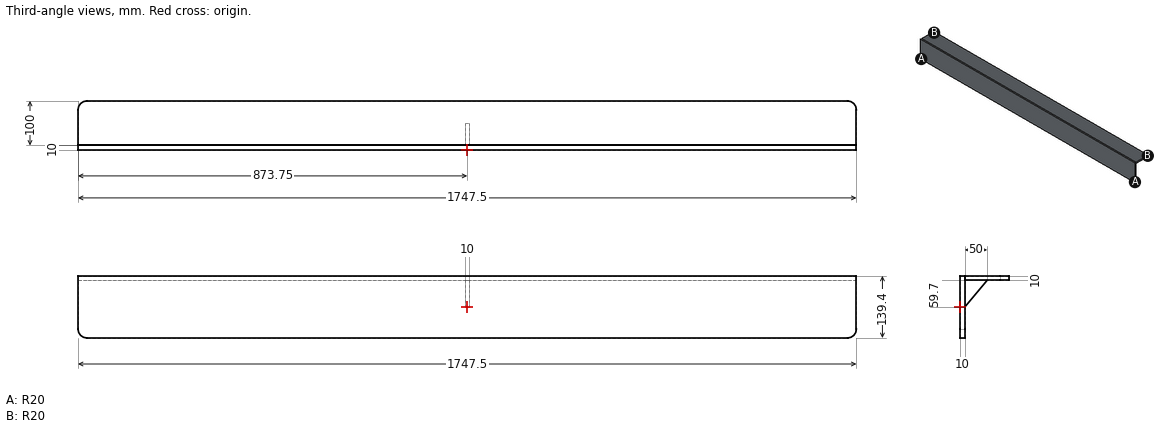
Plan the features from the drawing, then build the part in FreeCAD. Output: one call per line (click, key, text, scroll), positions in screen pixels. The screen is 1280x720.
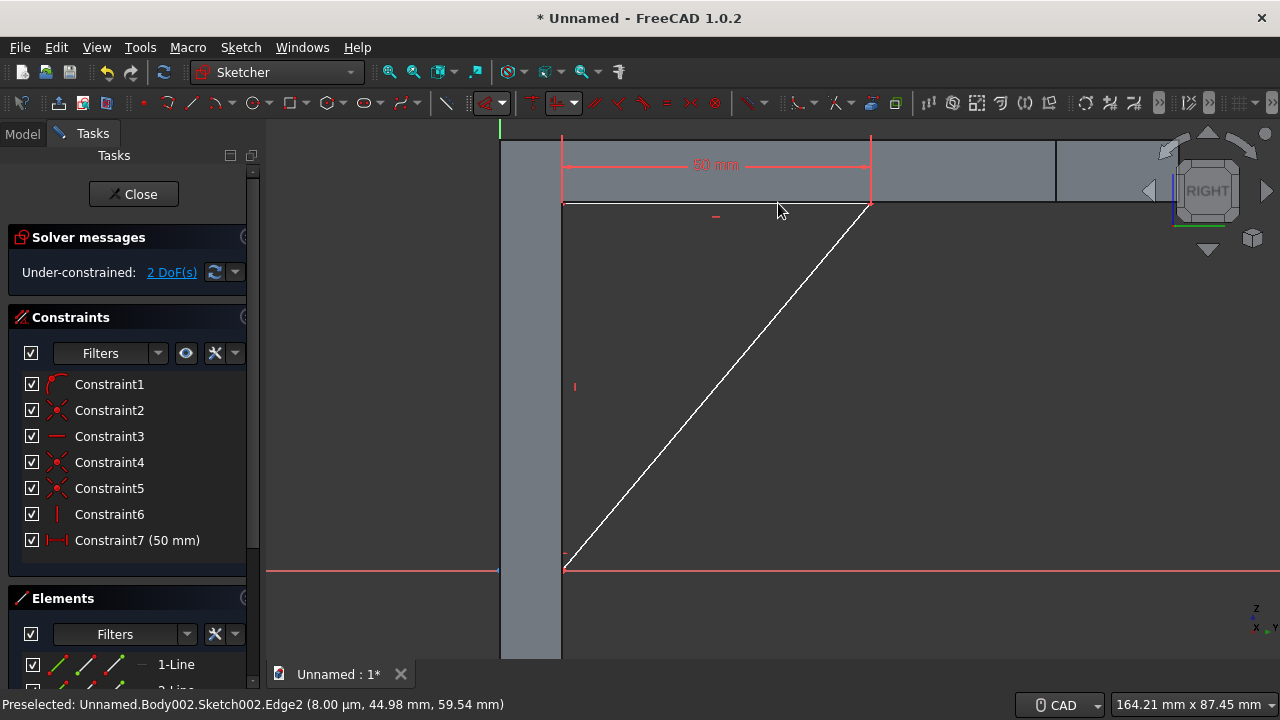
click(562, 571)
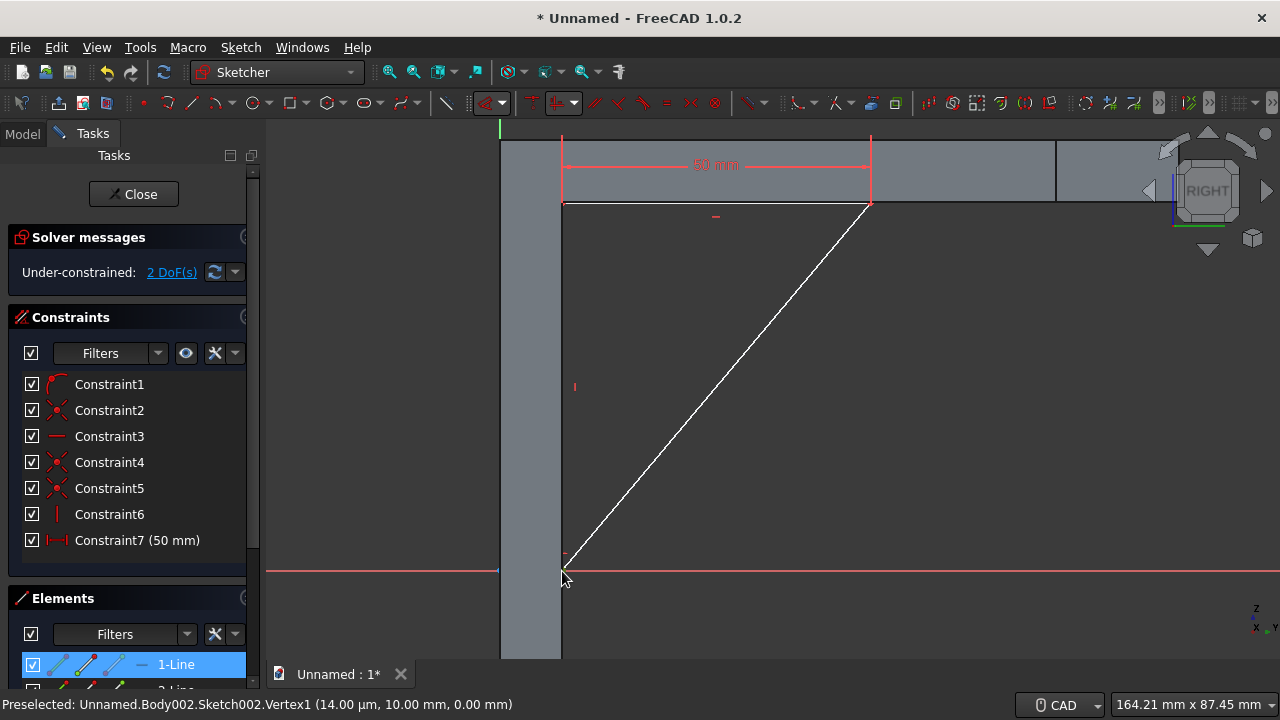
key(l)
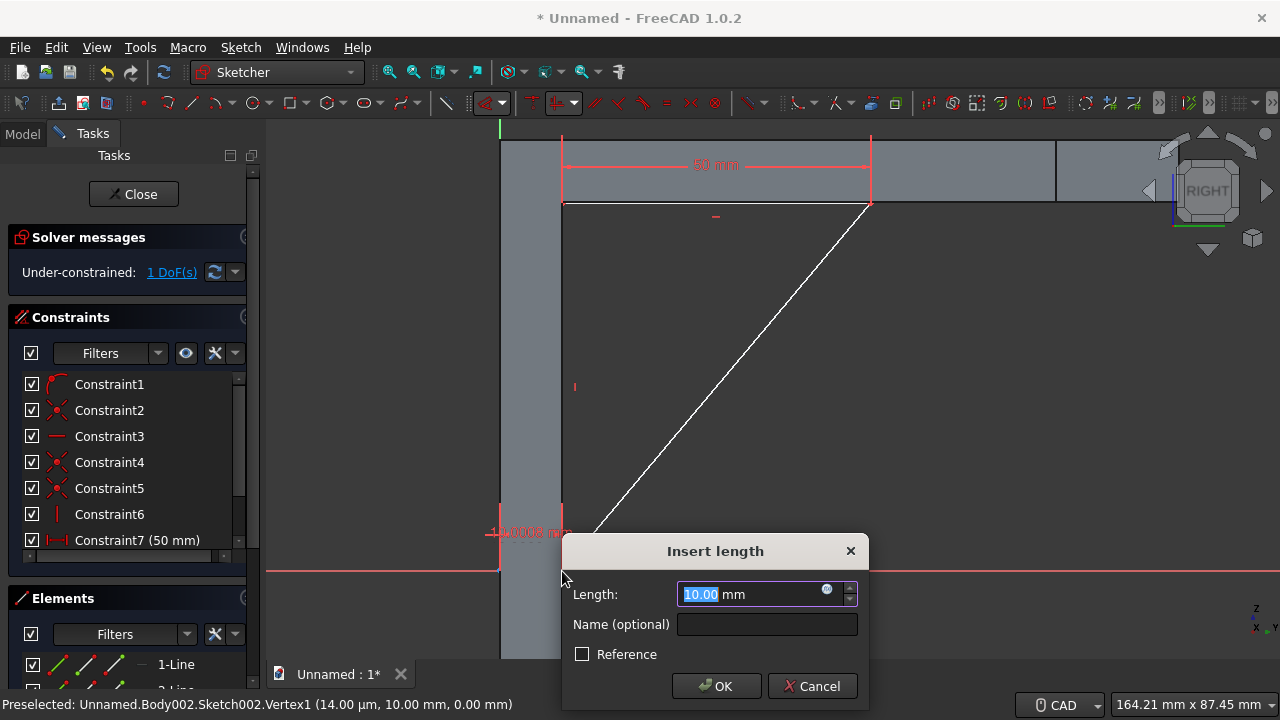
text(10)
key(Return)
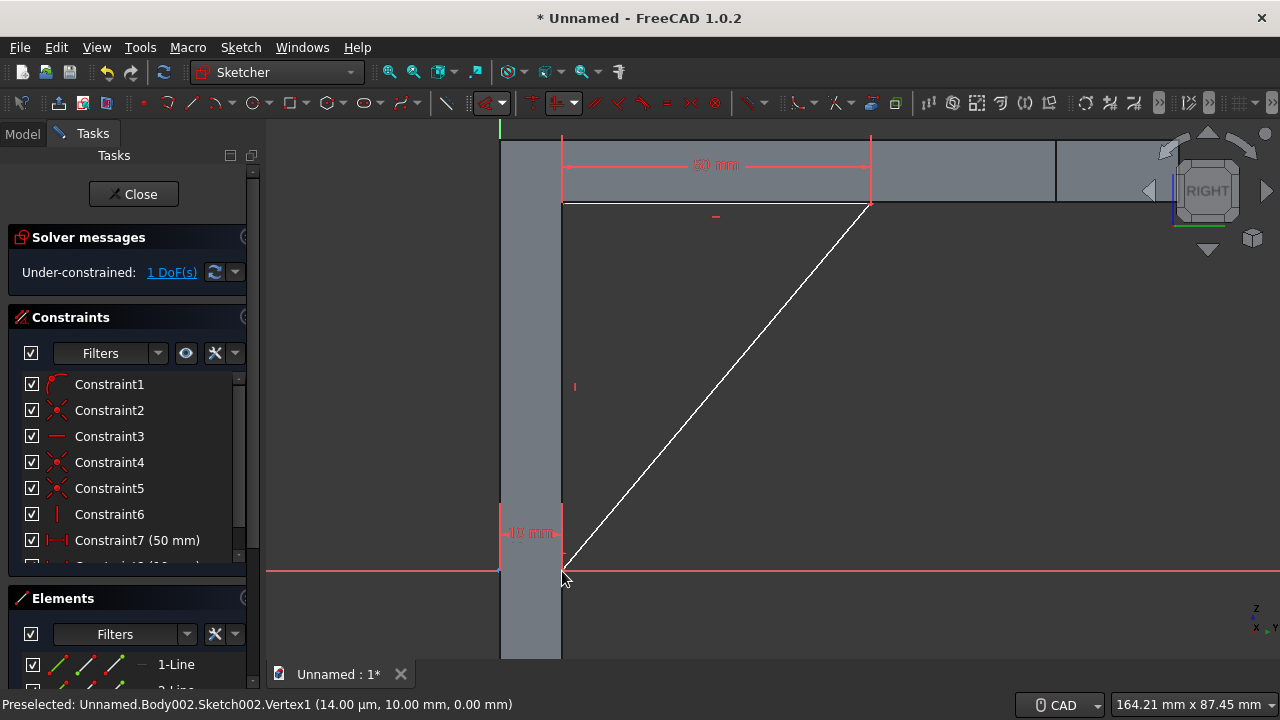
click(562, 313)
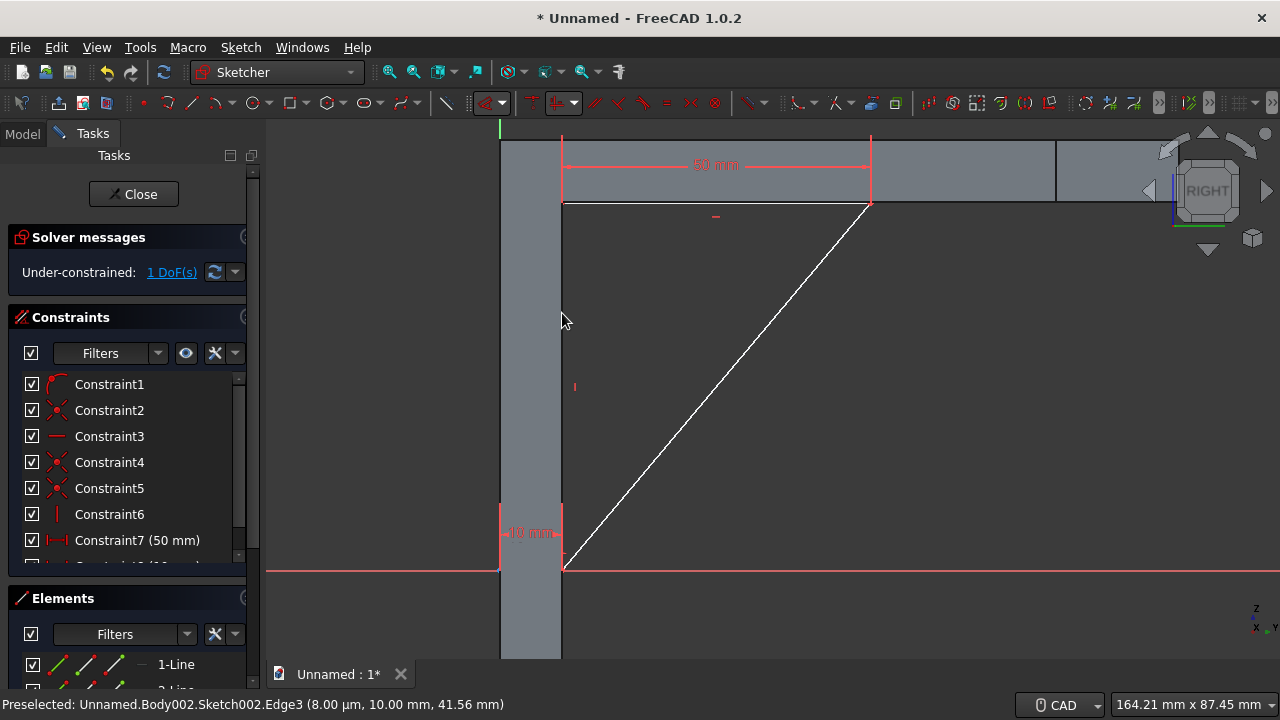
key(i)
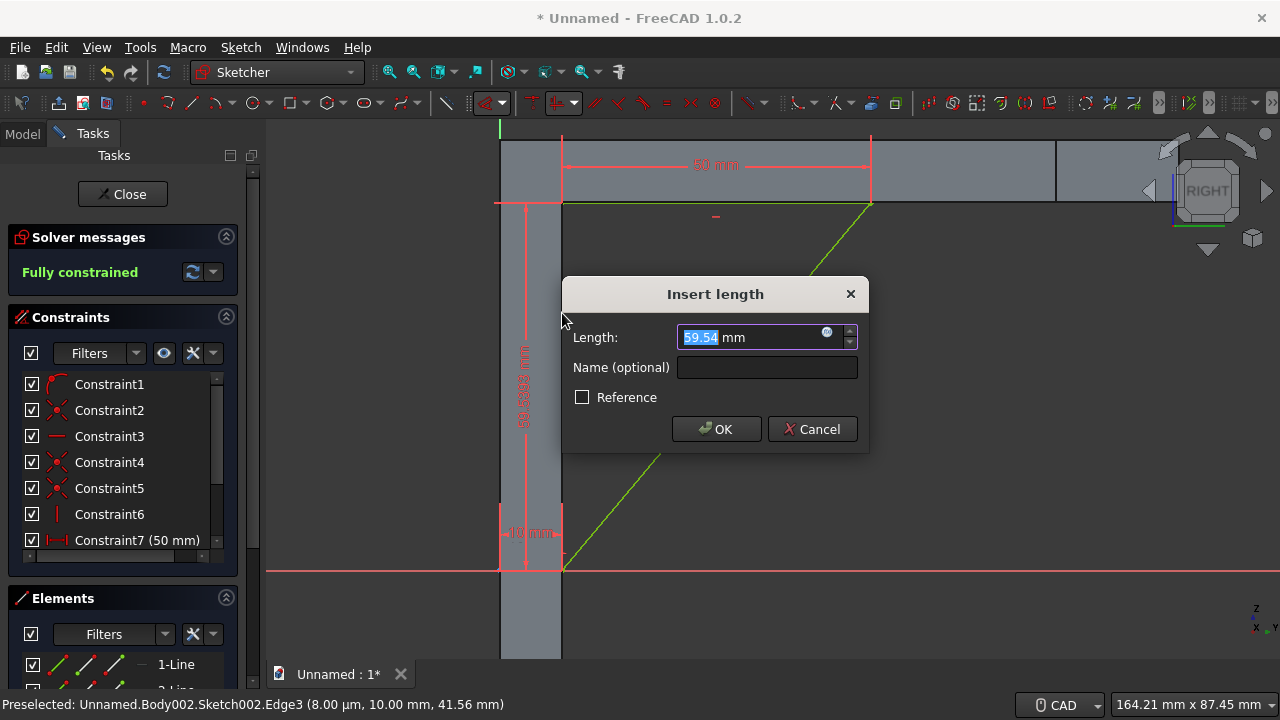
text(59.7)
key(Return)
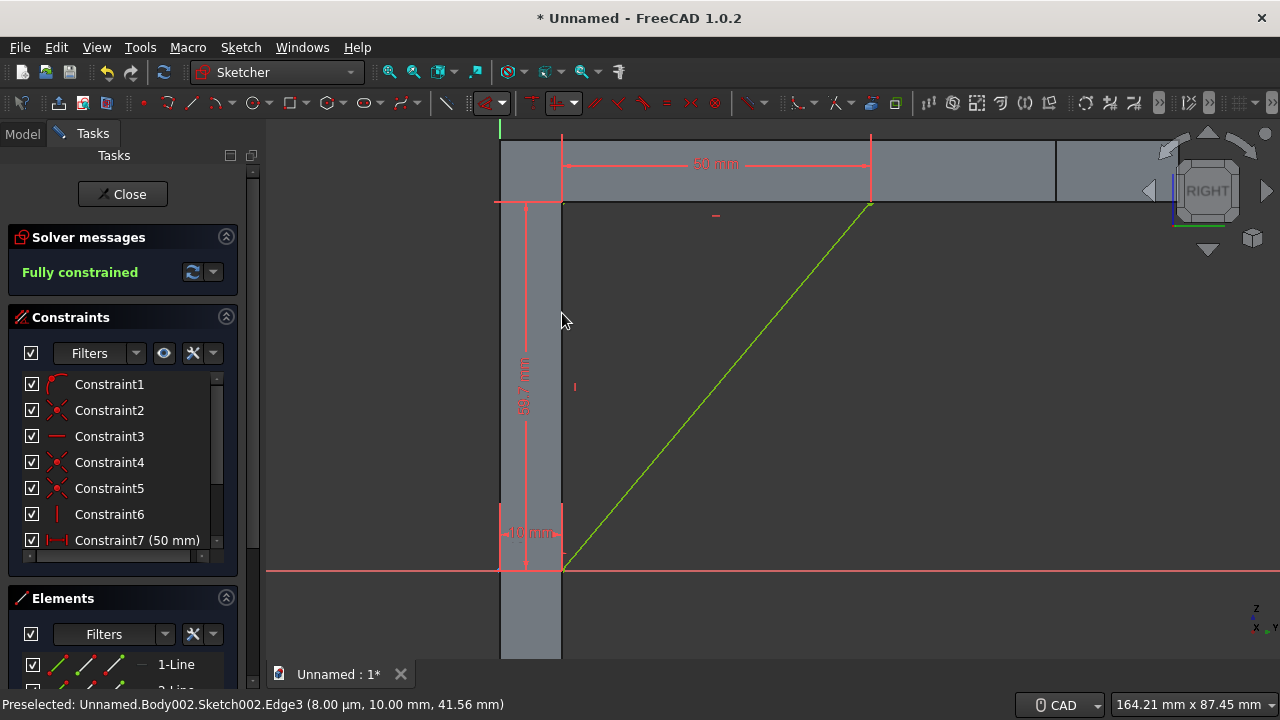
click(123, 194)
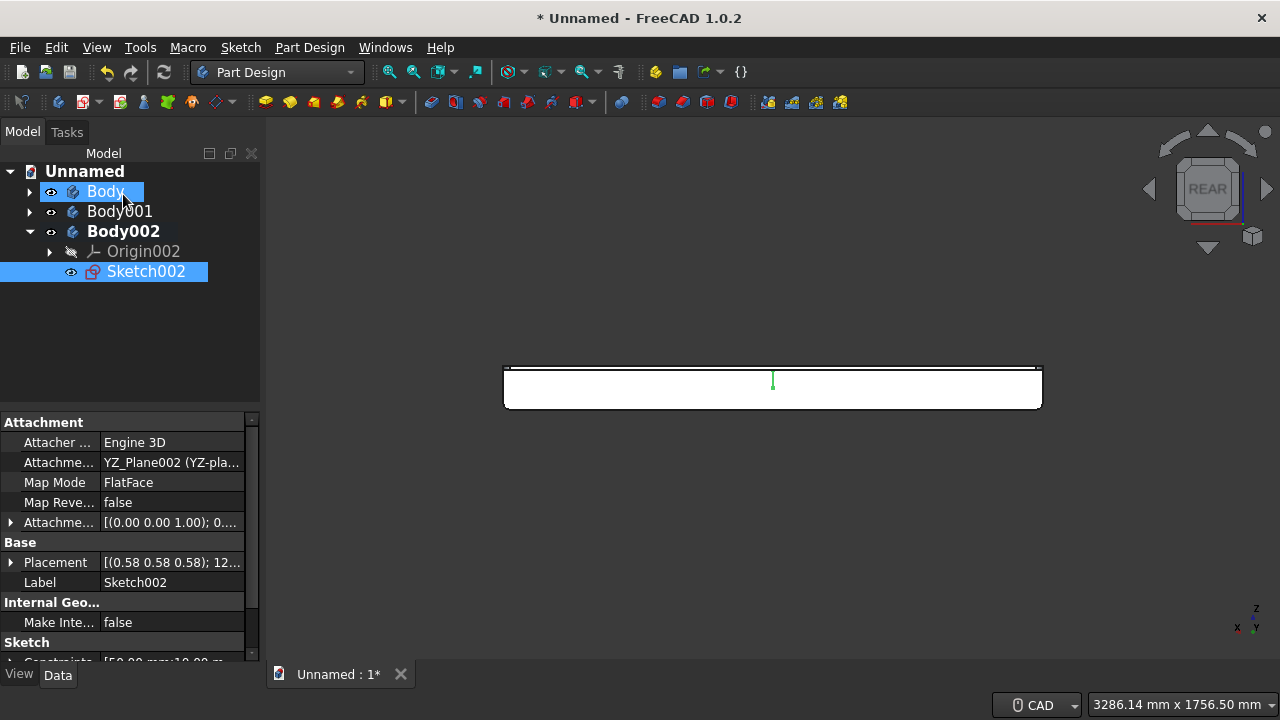
click(266, 102)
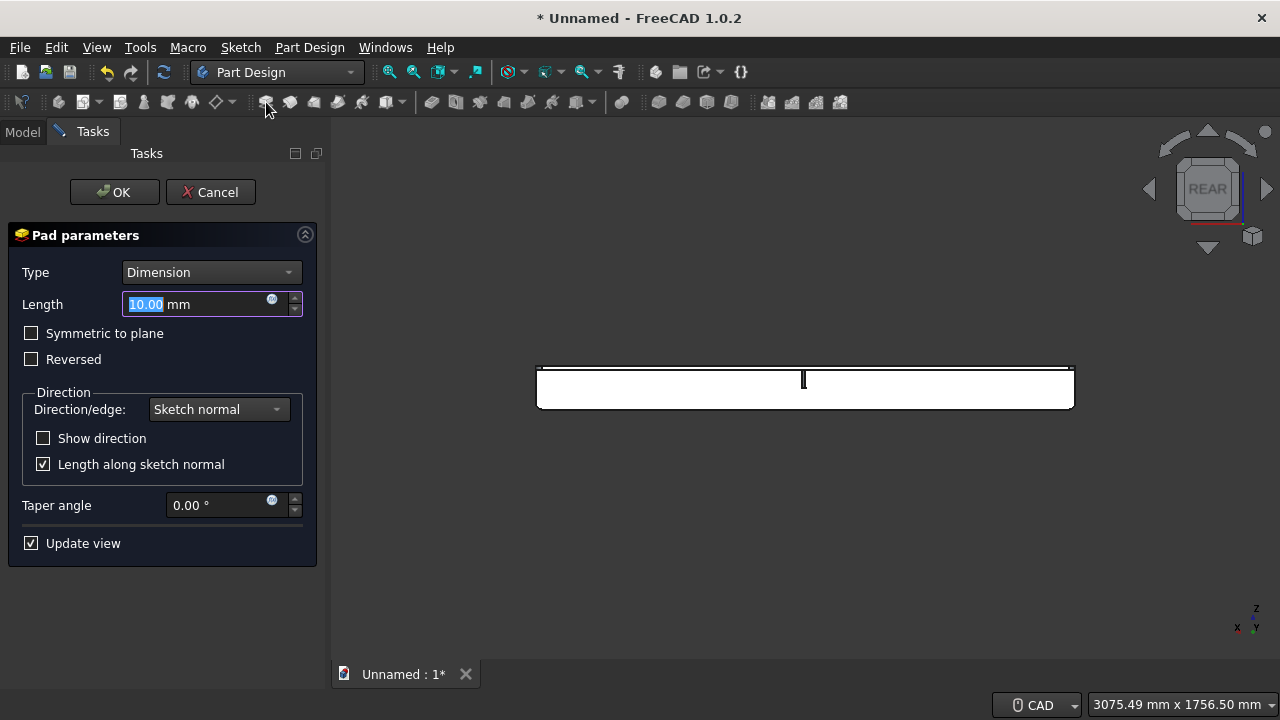
text(10)
key(Tab)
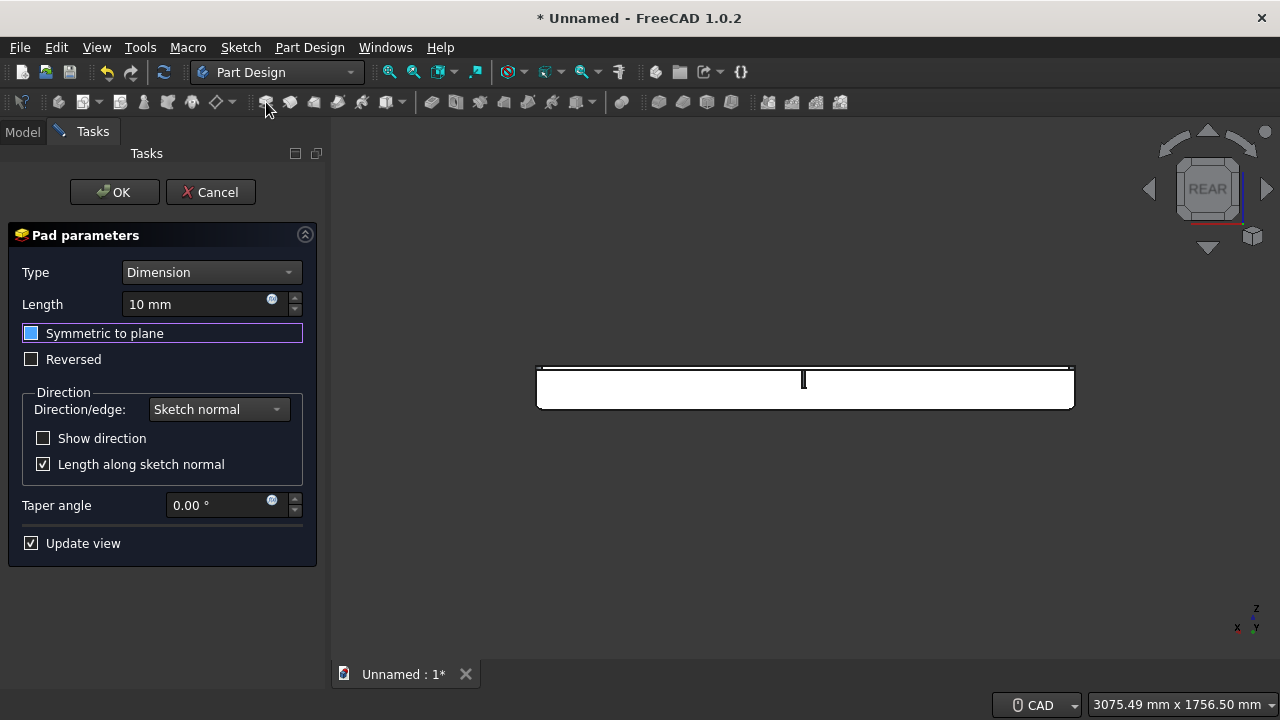
click(30, 333)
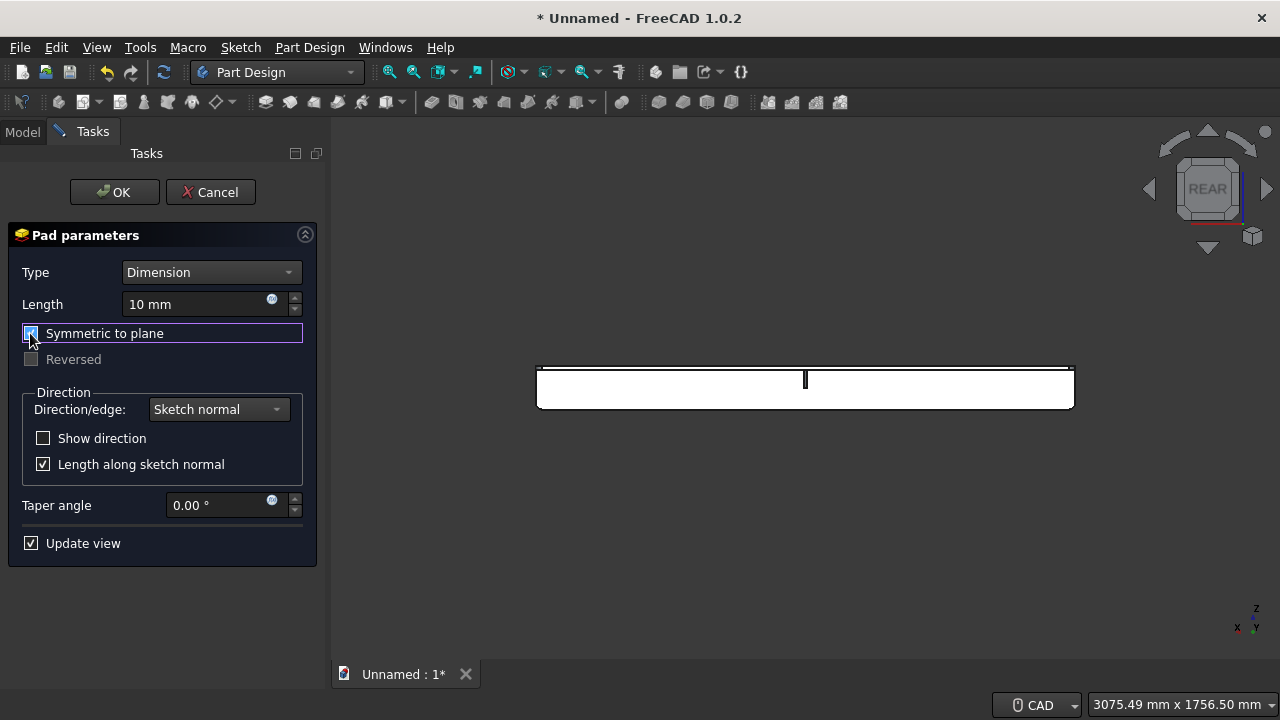
click(115, 192)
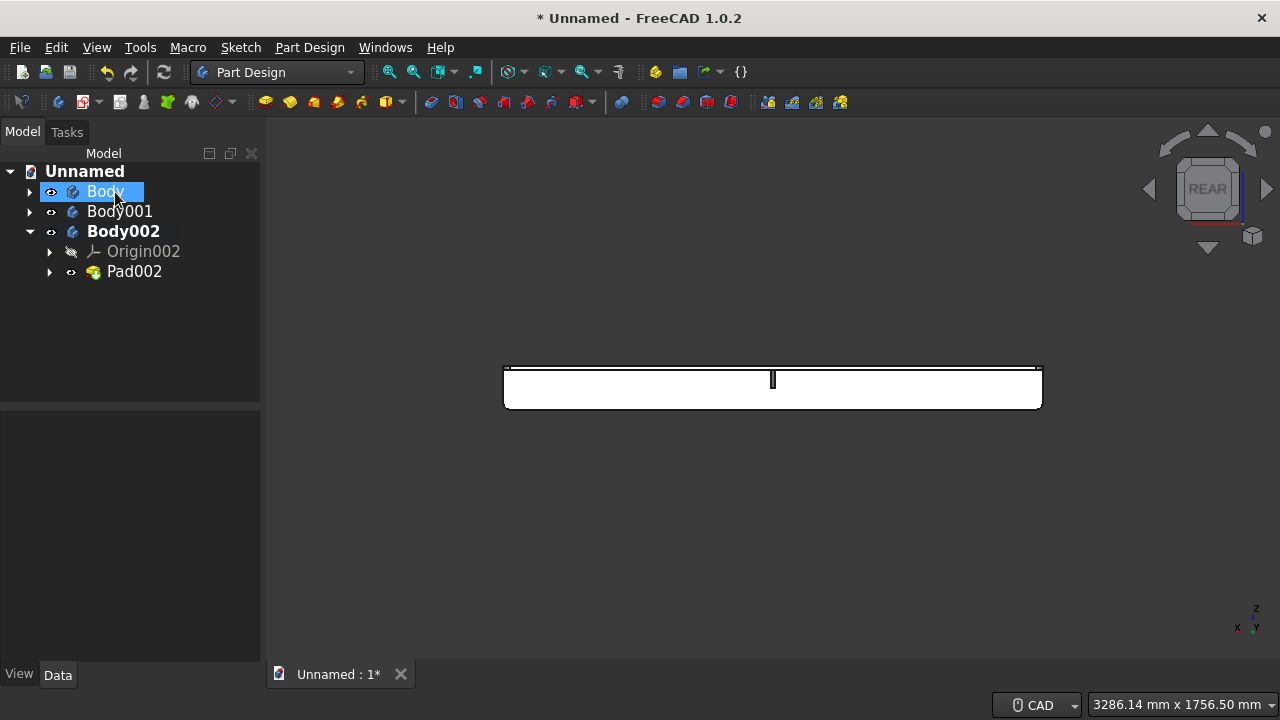
key(0)